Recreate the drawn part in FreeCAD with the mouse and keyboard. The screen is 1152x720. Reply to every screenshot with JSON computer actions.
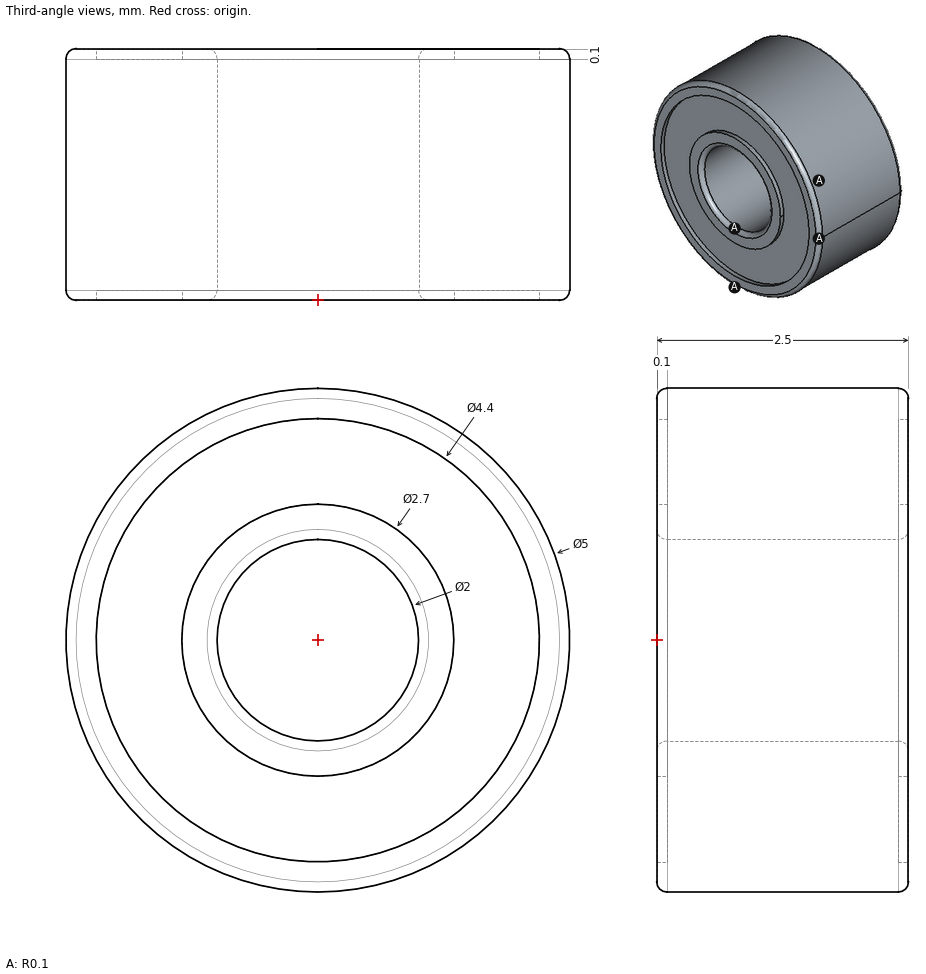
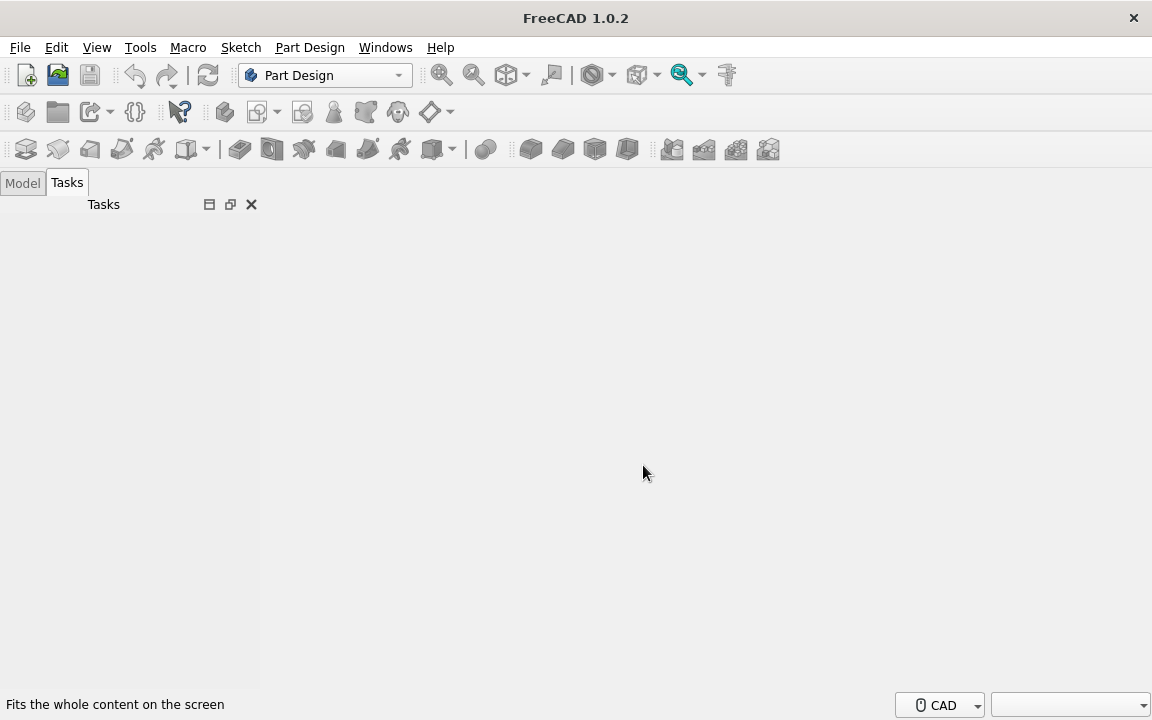
{"action": "left_click", "coordinate": [26, 76]}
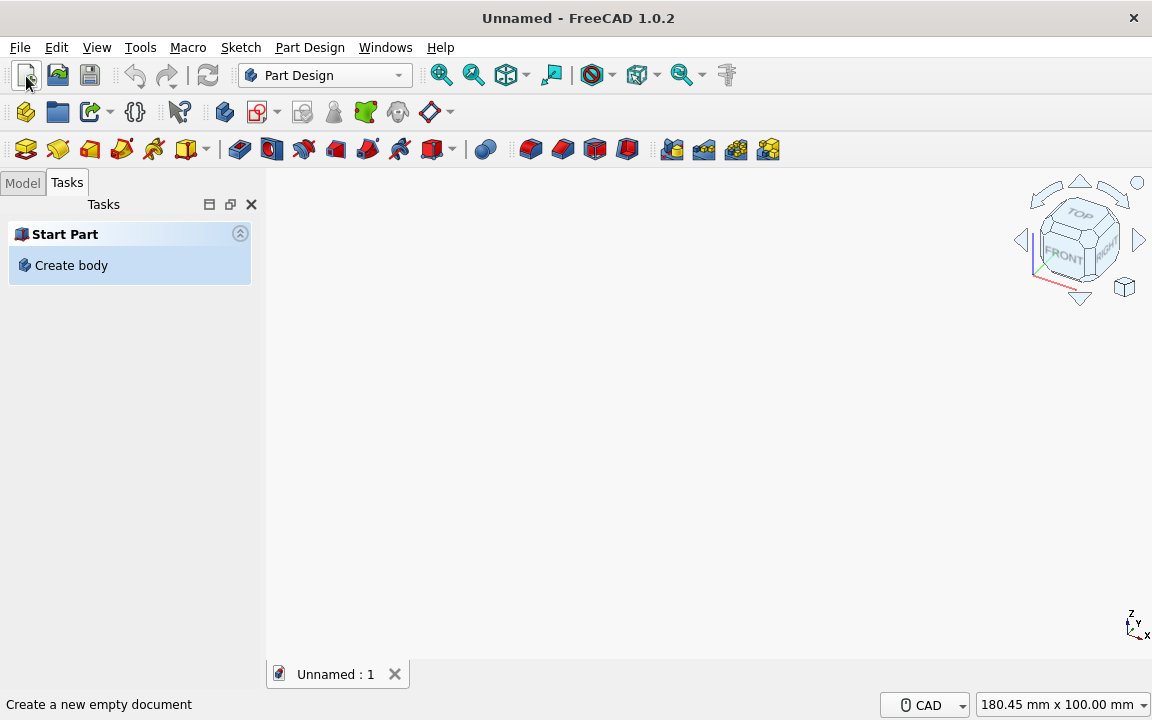
{"action": "left_click", "coordinate": [258, 112]}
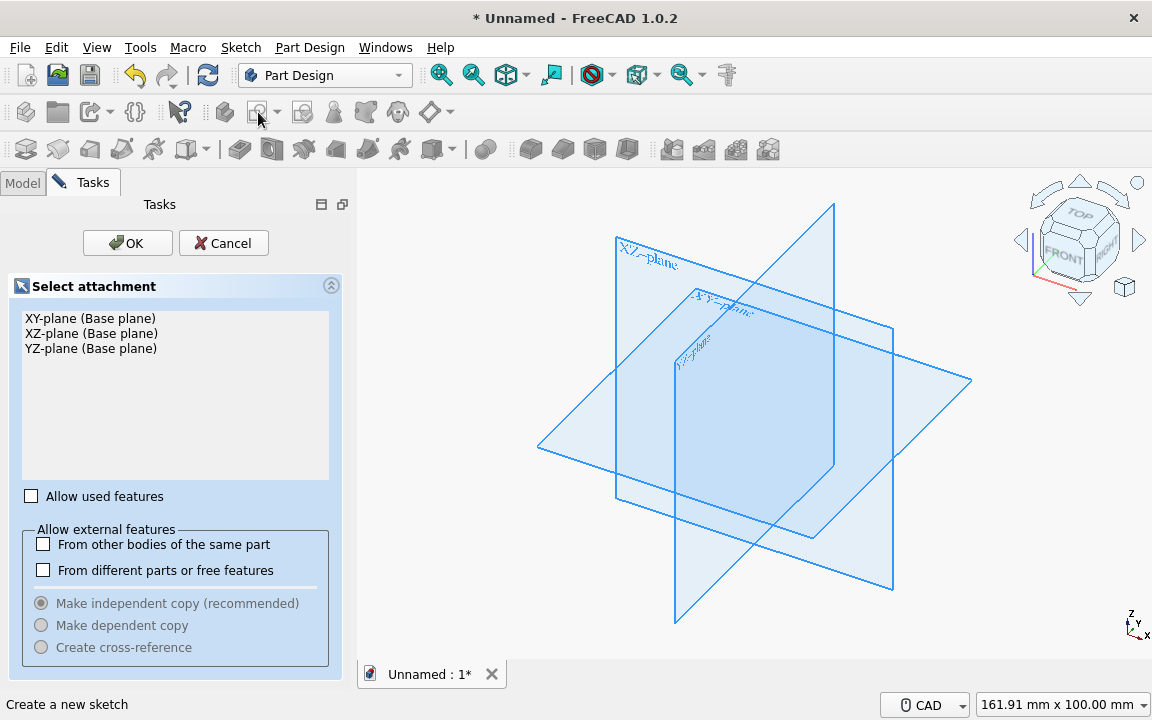
{"action": "left_click", "coordinate": [82, 334]}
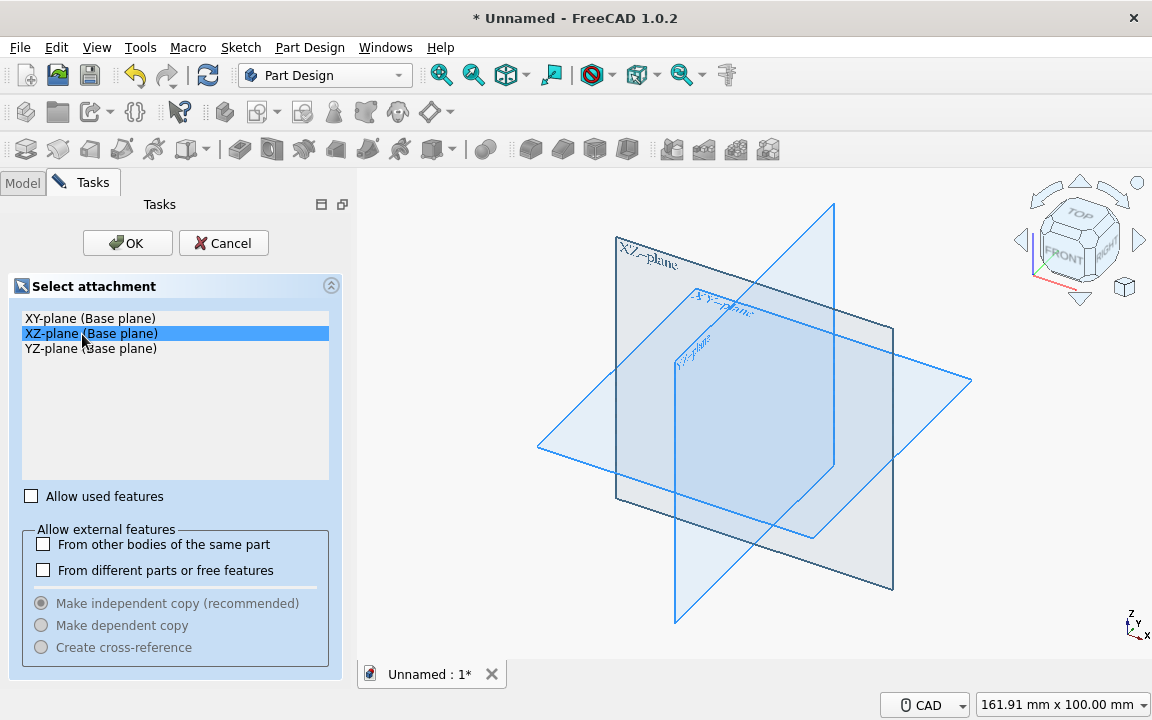
{"action": "left_click", "coordinate": [128, 243]}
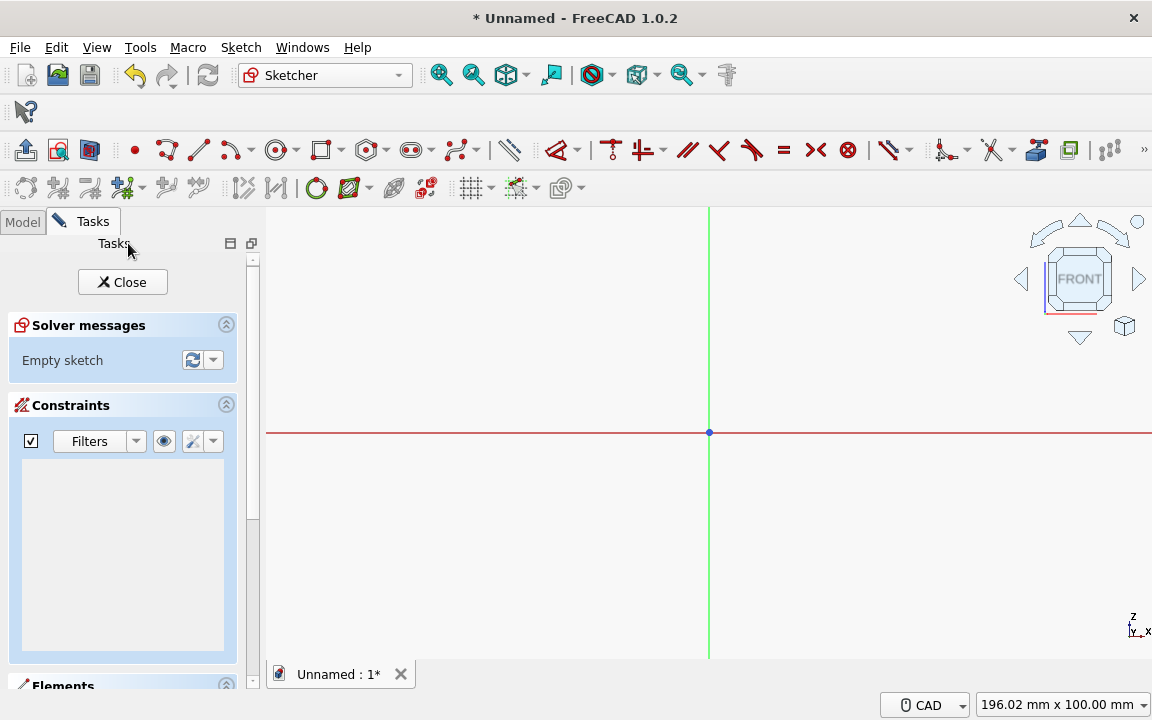
{"action": "scroll", "coordinate": [714, 433], "scroll_direction": "up", "scroll_amount": 13}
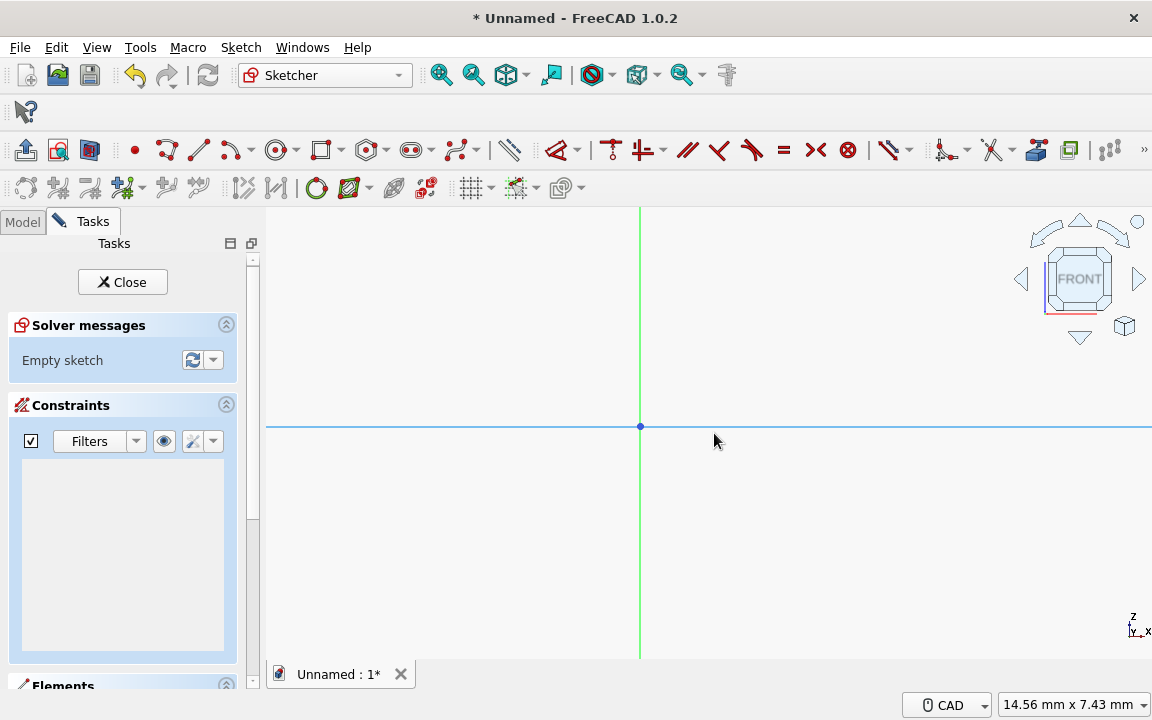
{"action": "left_click", "coordinate": [276, 150]}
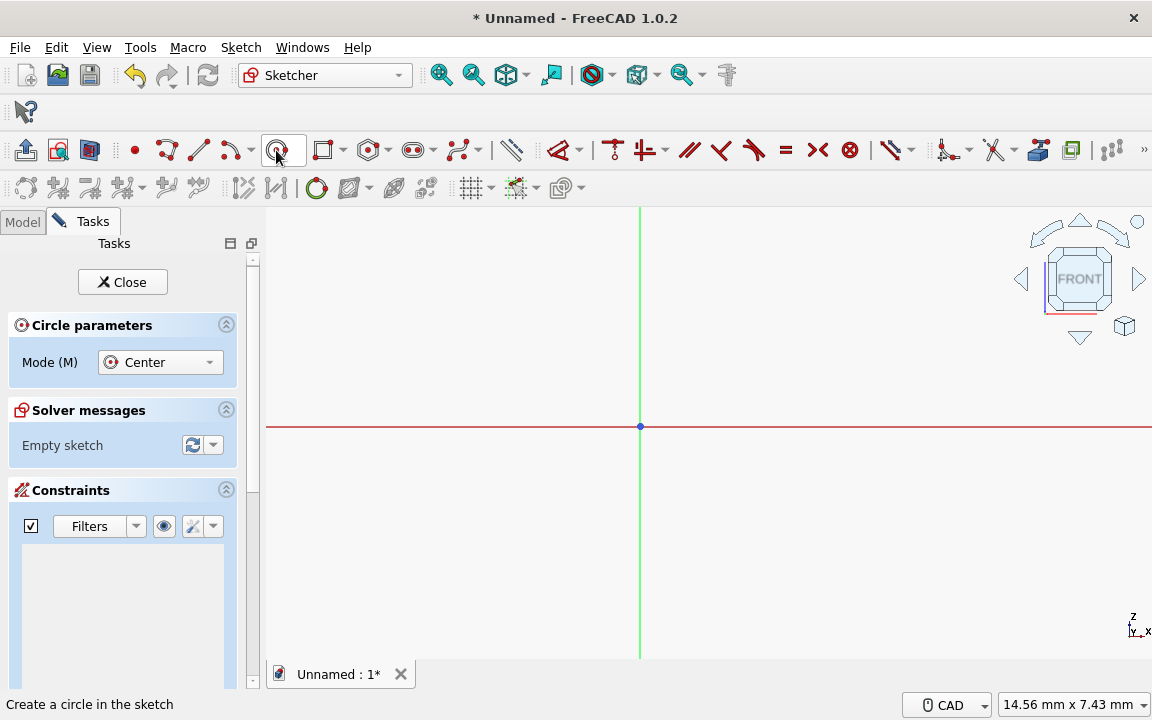
{"action": "left_click", "coordinate": [640, 427]}
{"action": "mouse_move", "coordinate": [748, 319]}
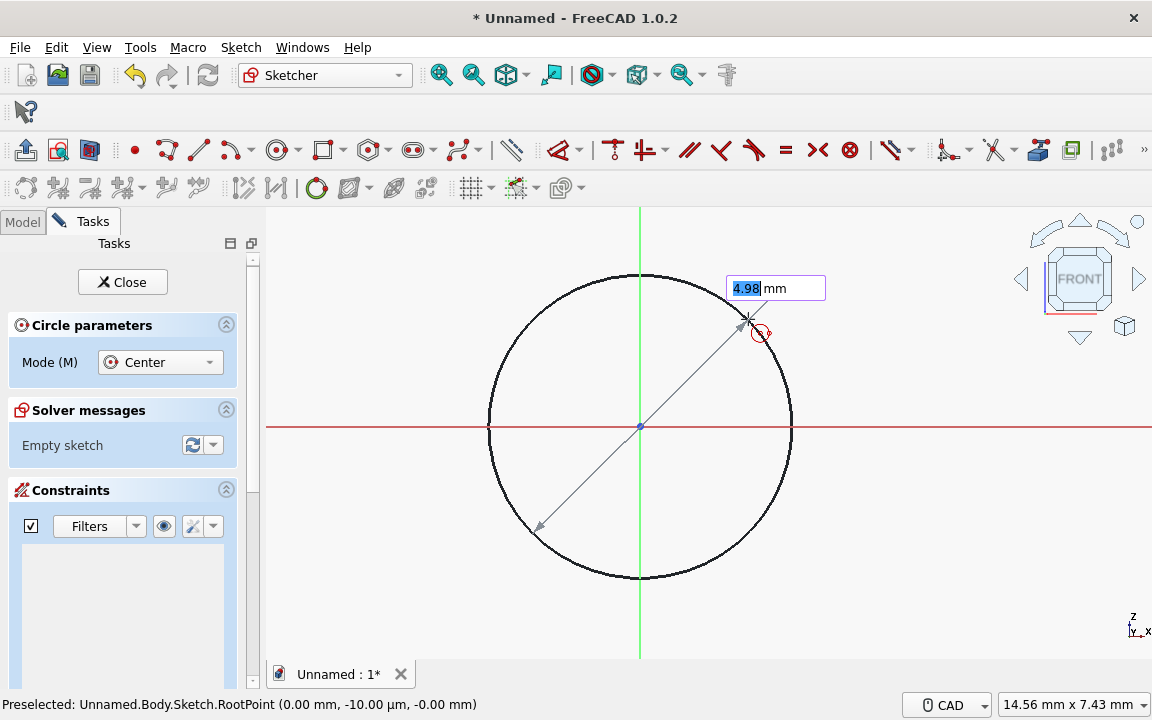
{"action": "type", "text": "5"}
{"action": "key", "text": "Return"}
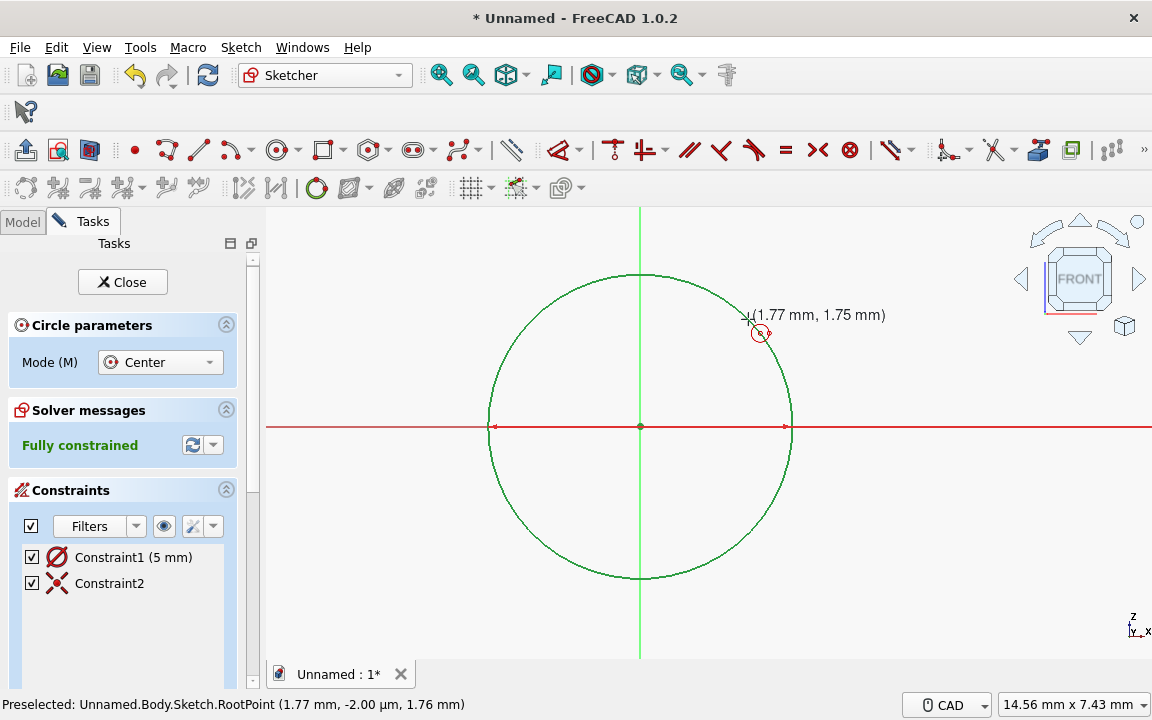
{"action": "left_click", "coordinate": [640, 427]}
{"action": "mouse_move", "coordinate": [683, 384]}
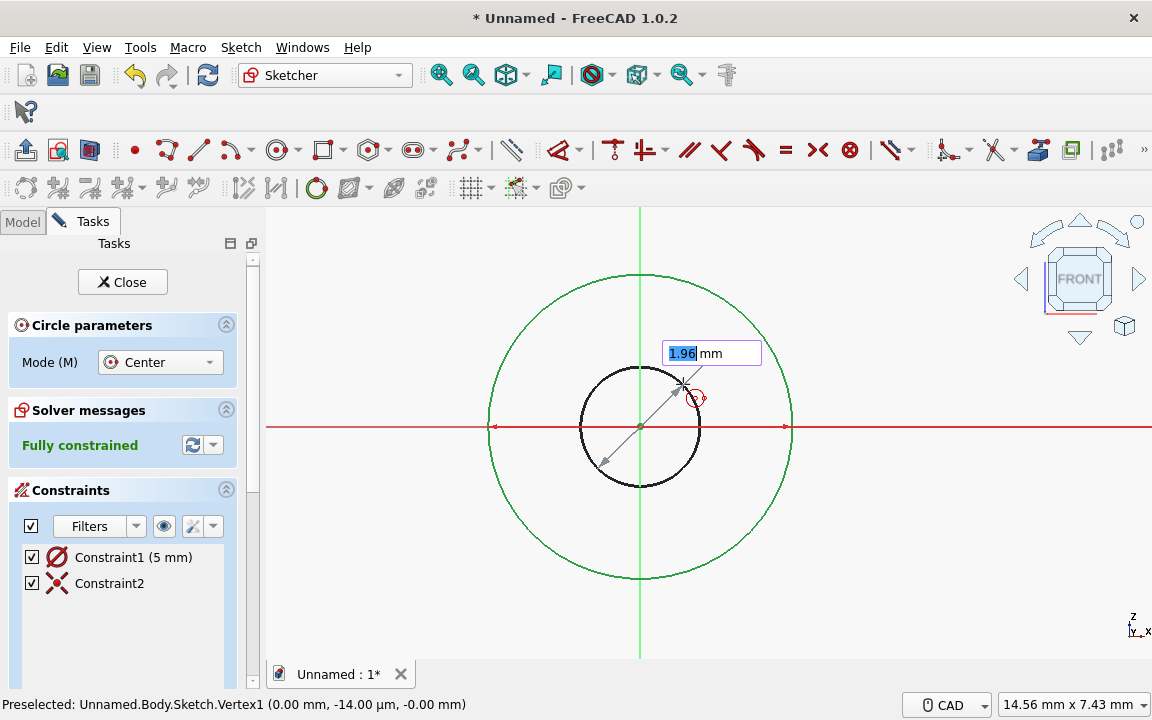
{"action": "type", "text": "2"}
{"action": "key", "text": "Return"}
{"action": "key", "text": "Escape"}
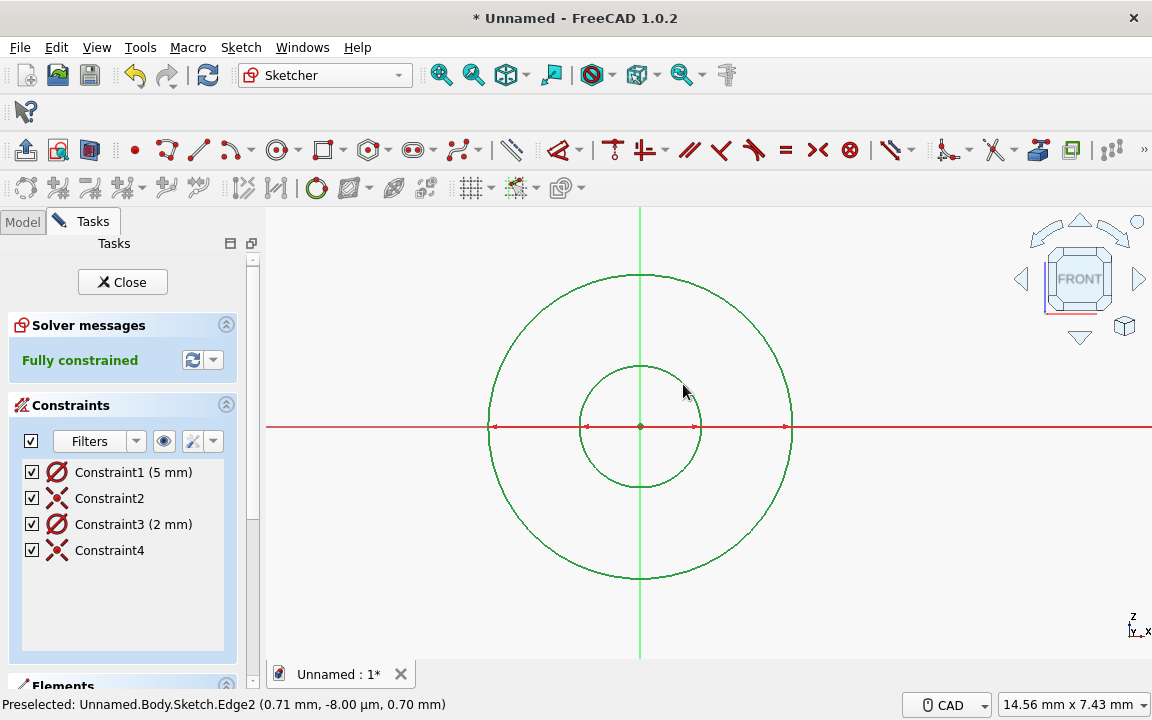
{"action": "left_click", "coordinate": [123, 282]}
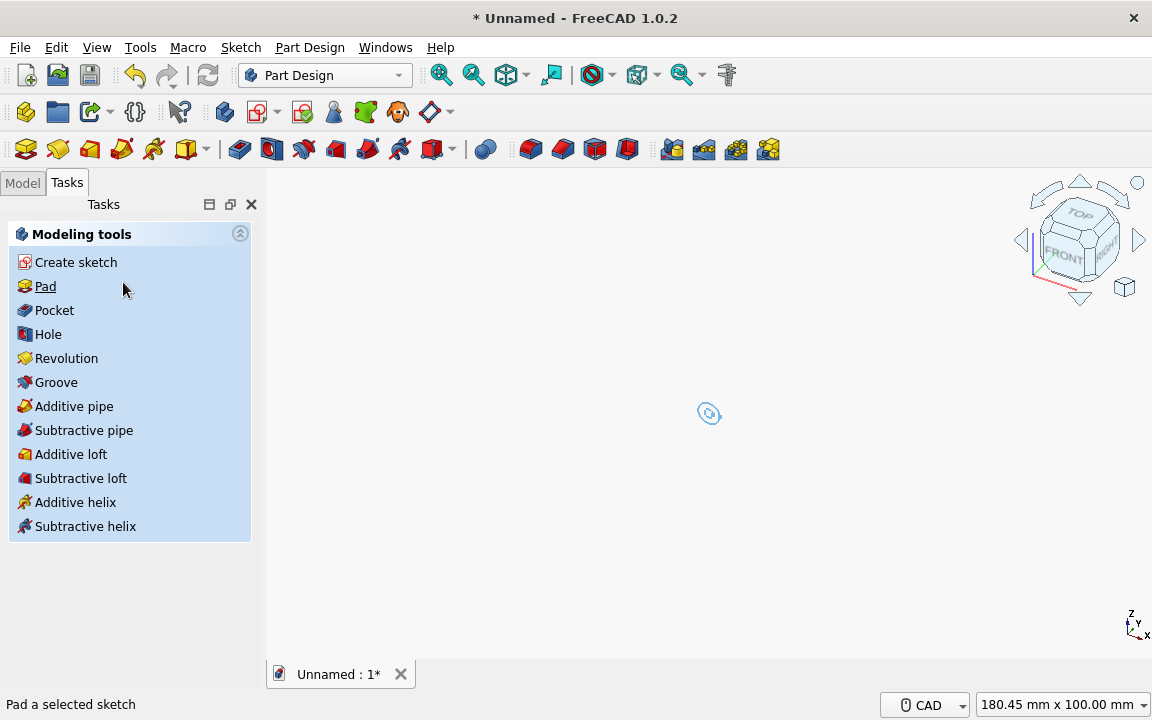
{"action": "left_click", "coordinate": [26, 150]}